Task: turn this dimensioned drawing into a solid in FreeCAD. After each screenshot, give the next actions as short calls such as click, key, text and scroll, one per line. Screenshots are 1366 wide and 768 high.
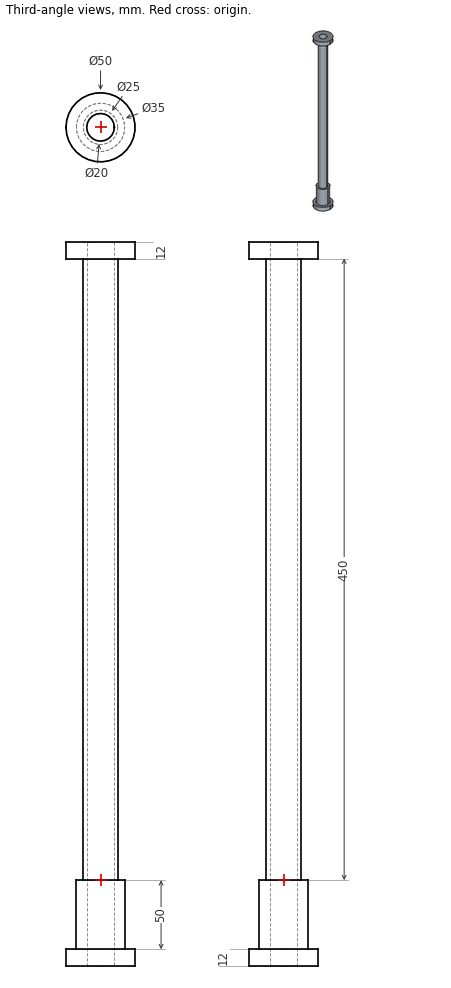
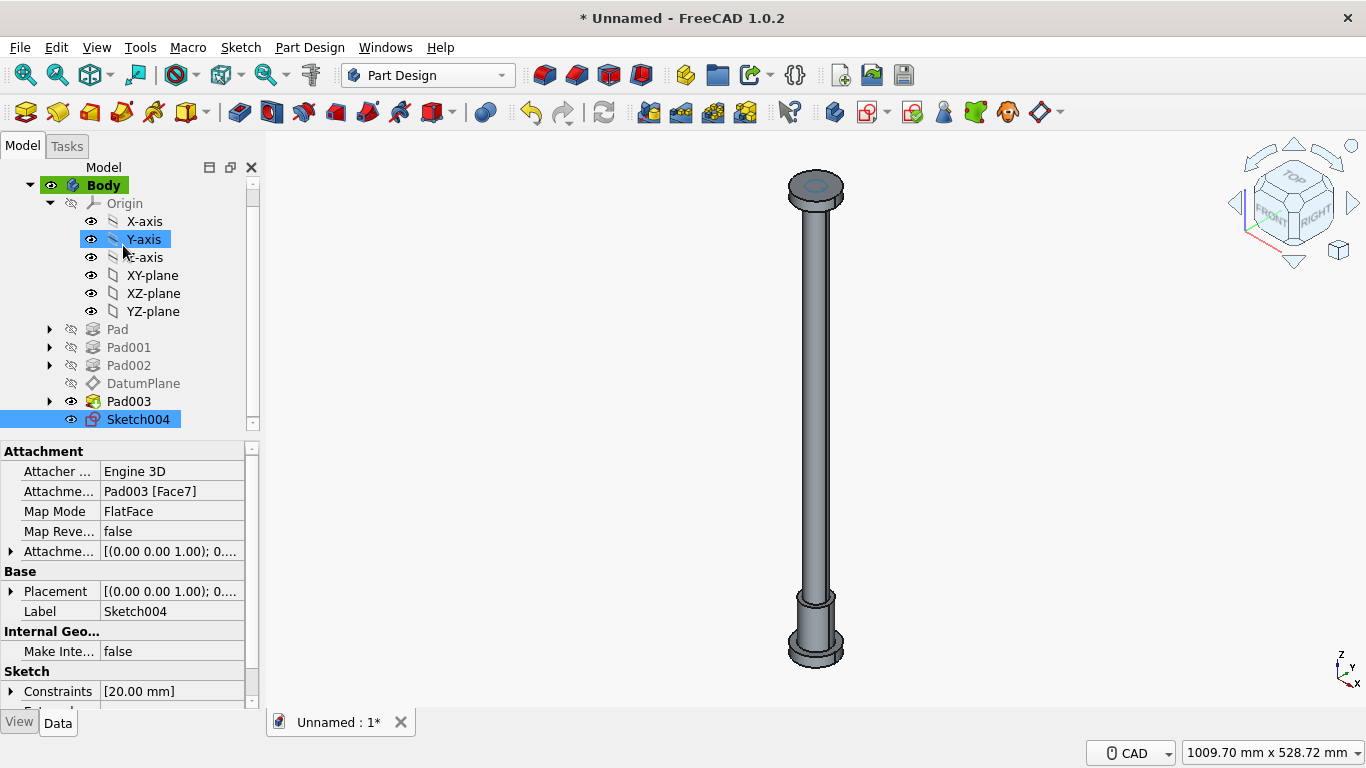
click(240, 112)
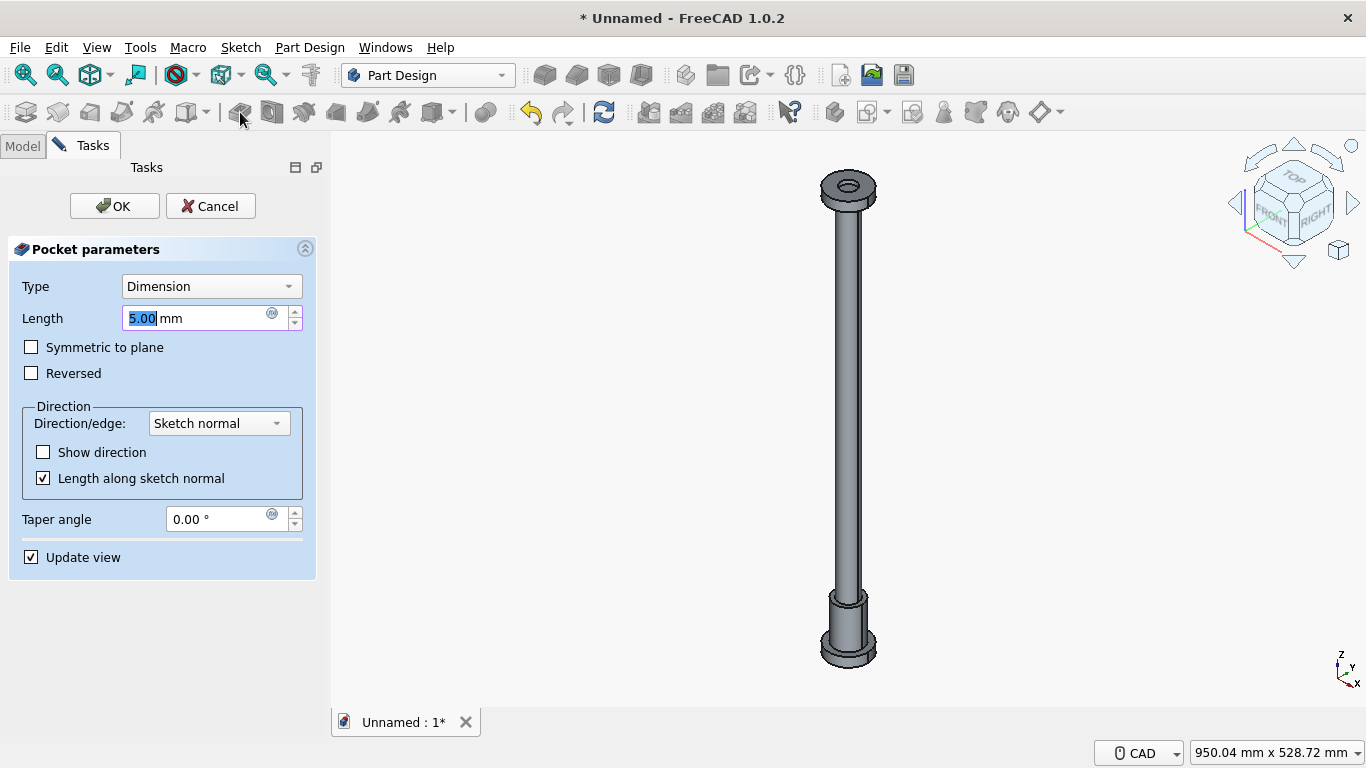
click(212, 286)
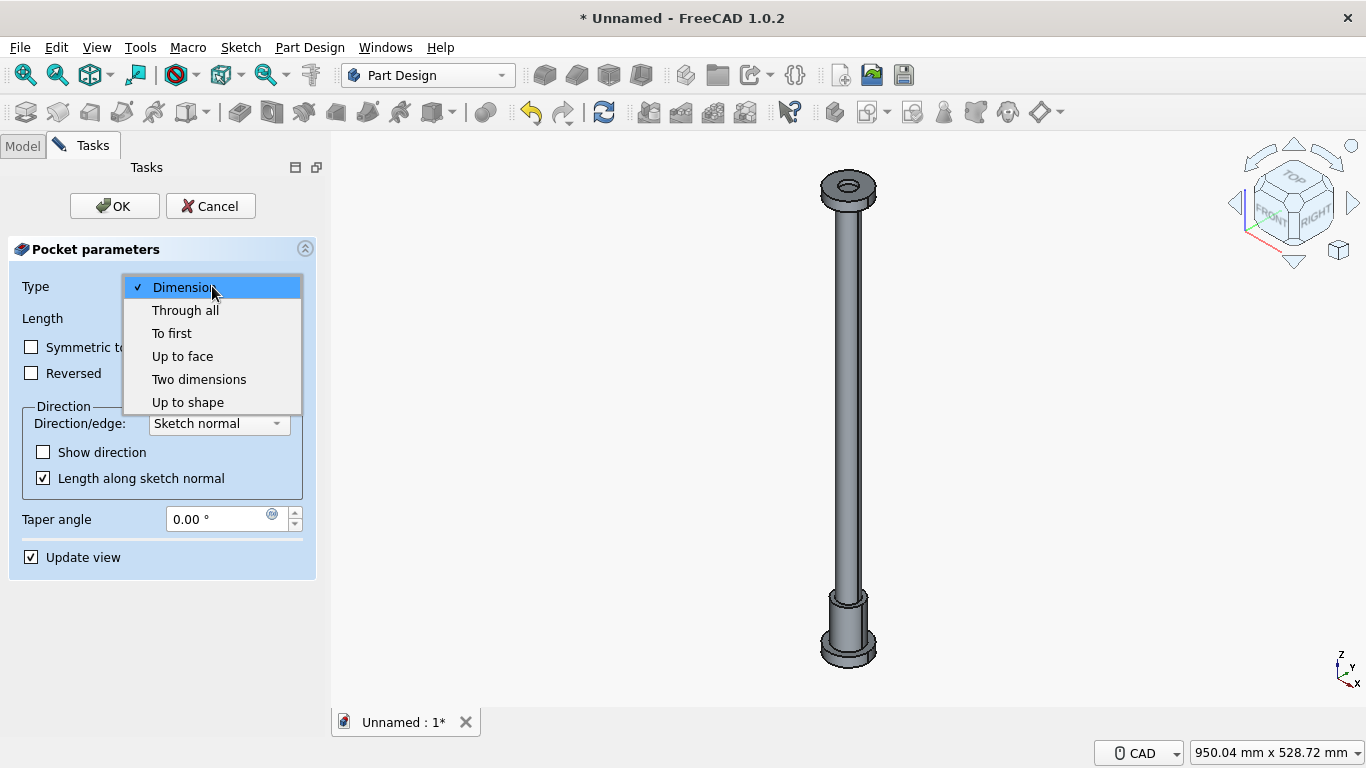
click(212, 310)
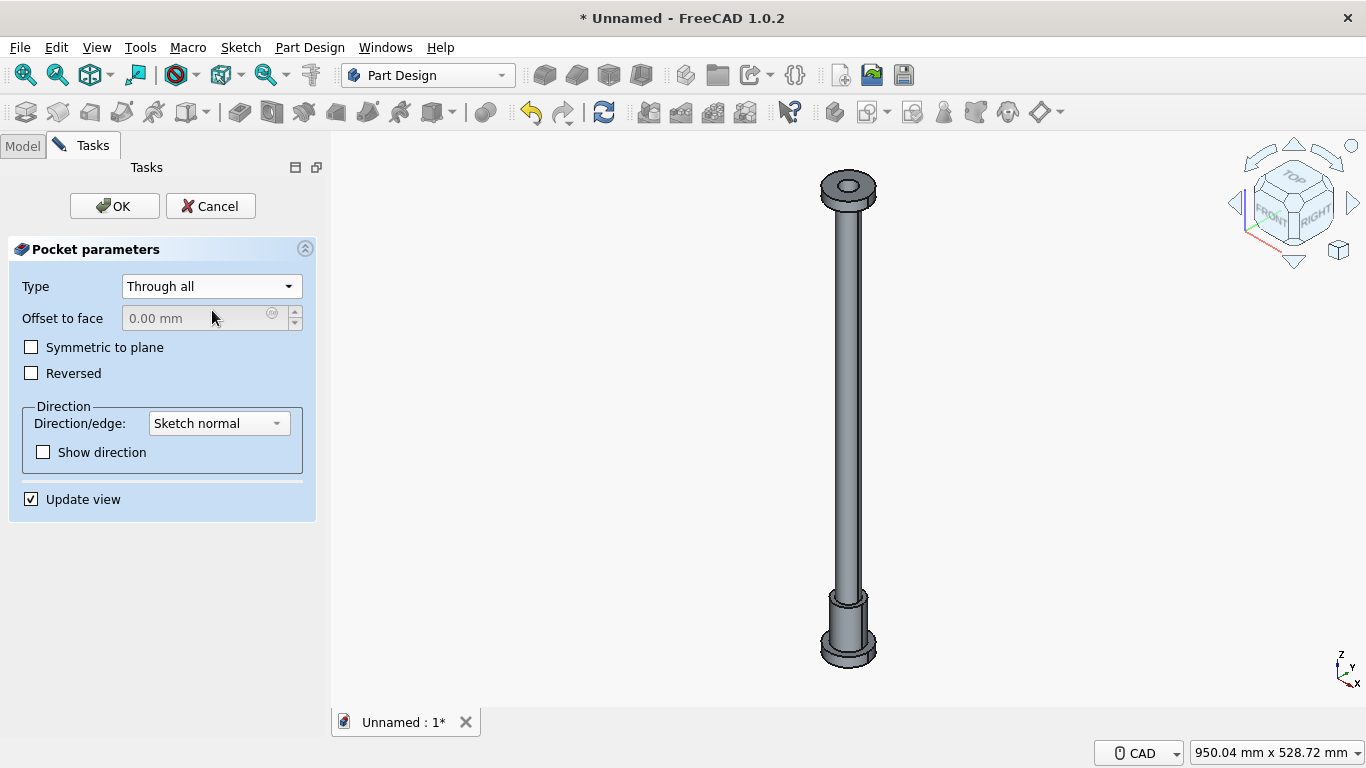
click(115, 206)